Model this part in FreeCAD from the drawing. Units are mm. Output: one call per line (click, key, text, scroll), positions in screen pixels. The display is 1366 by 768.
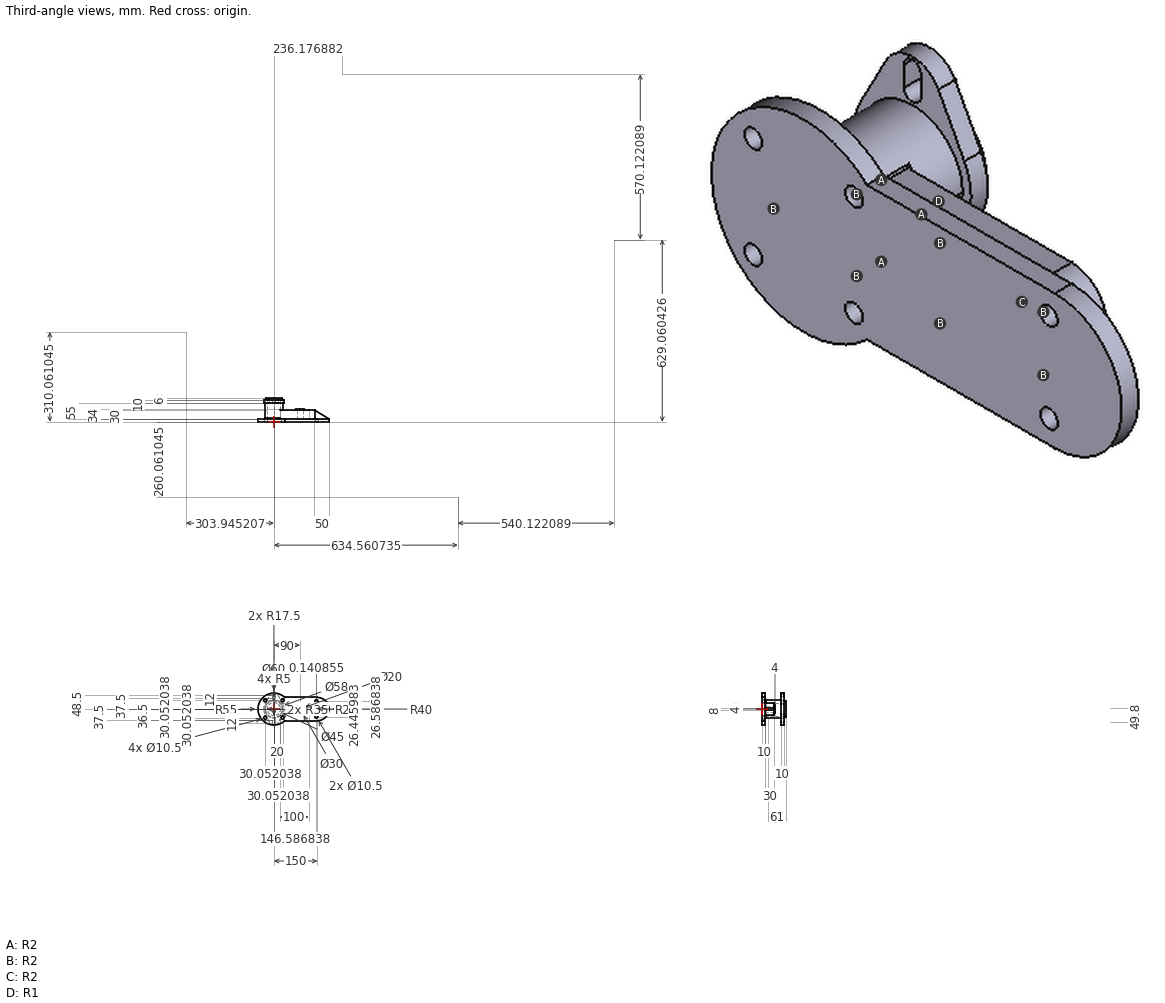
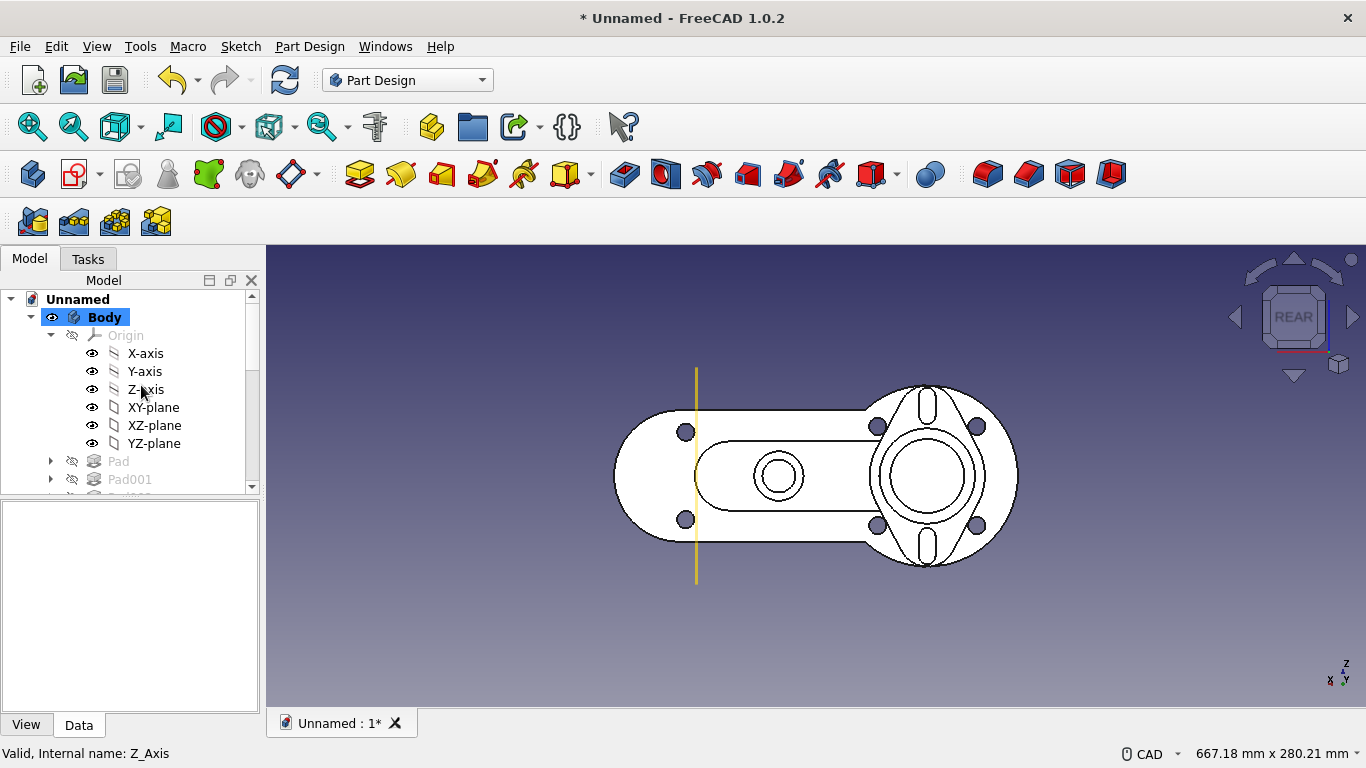
scroll(101, 385, down, 6)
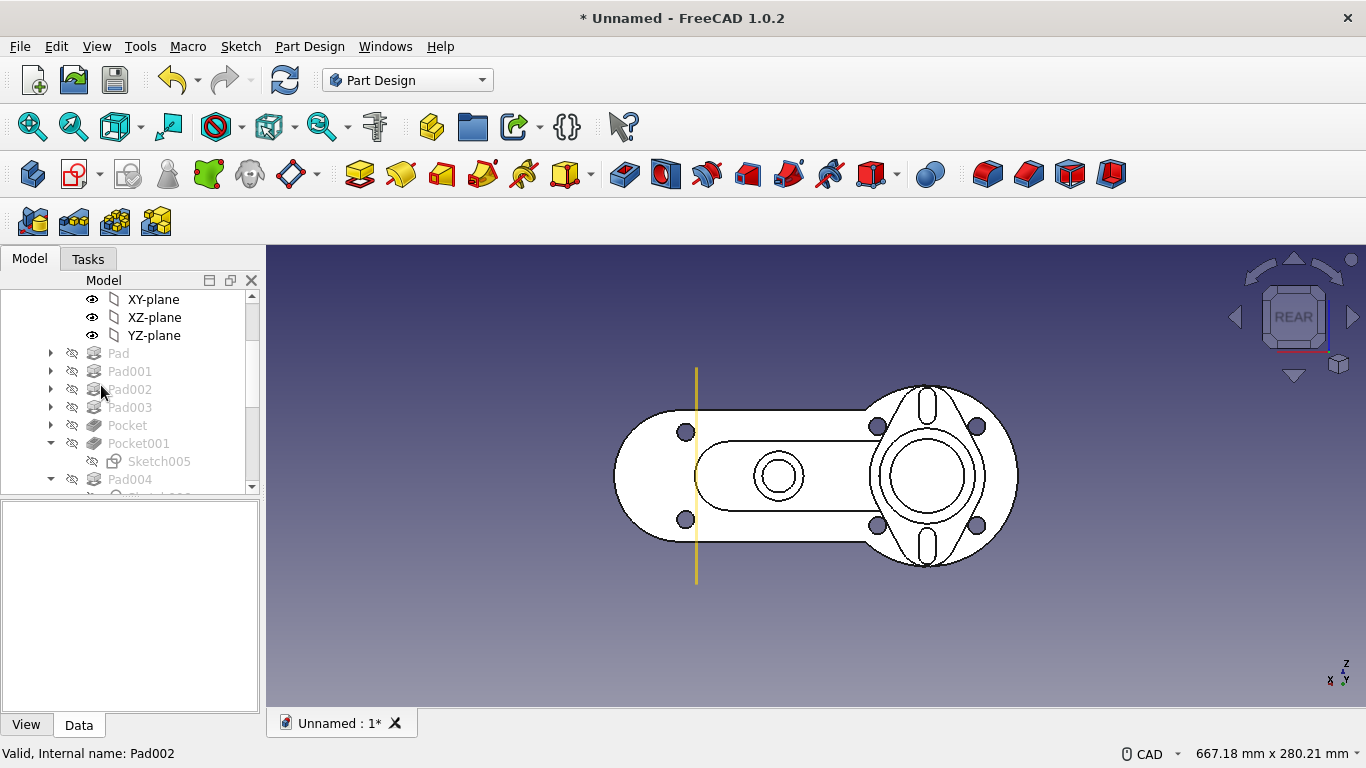
click(117, 479)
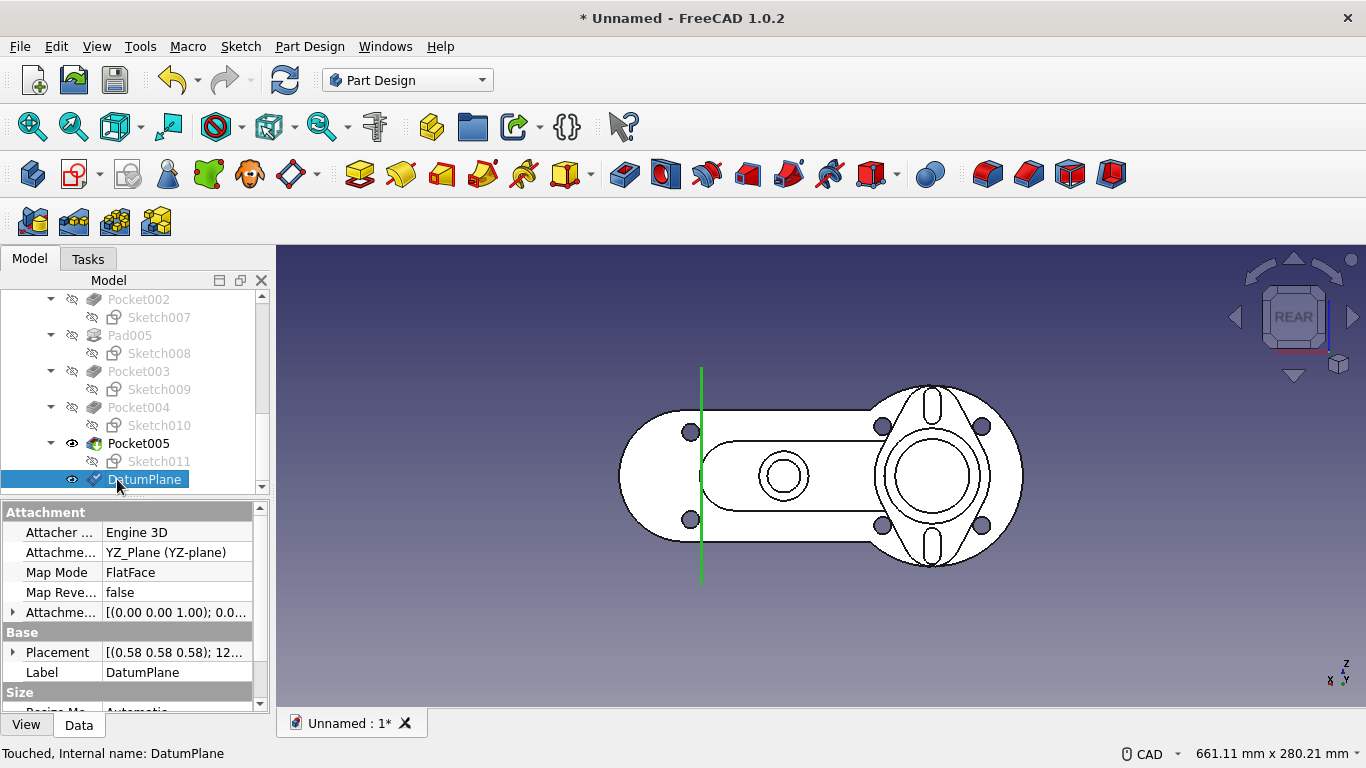
click(74, 174)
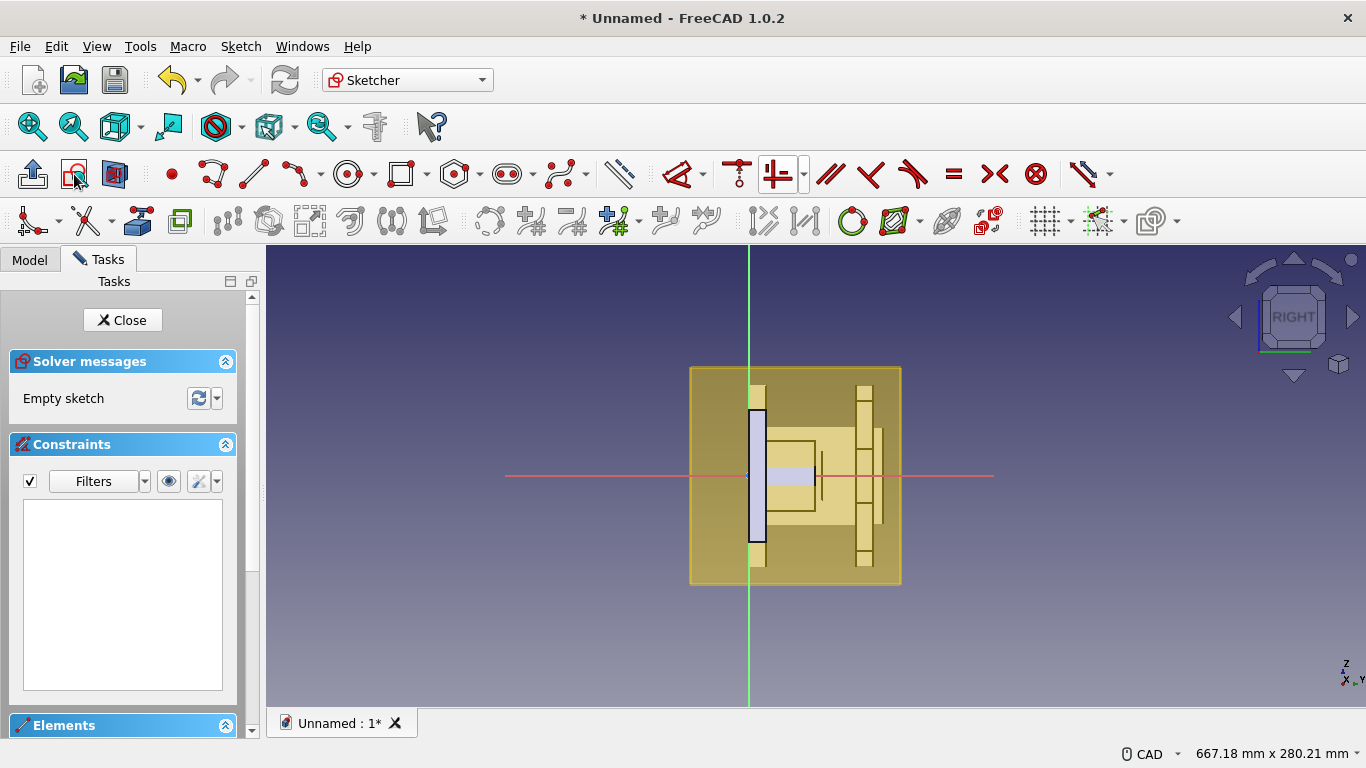
key(q)
key(s)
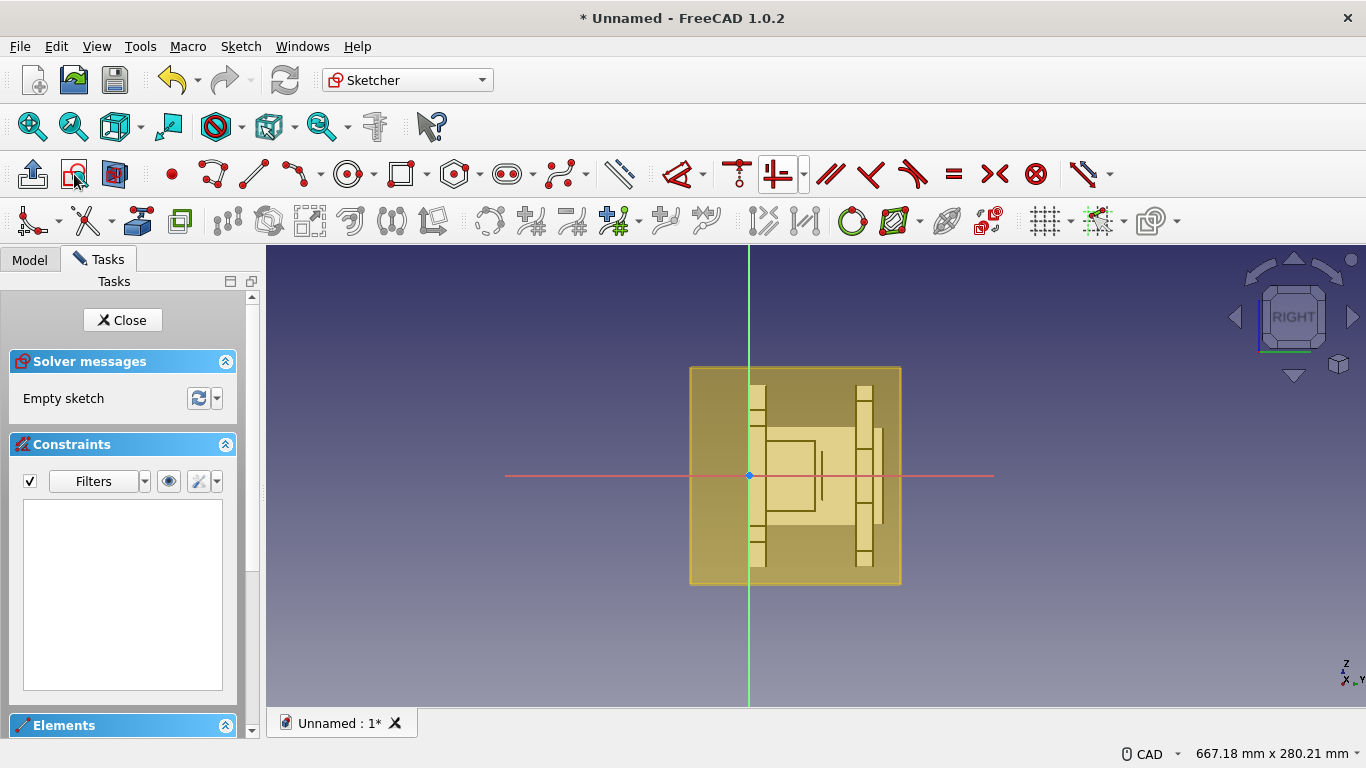
scroll(787, 476, up, 11)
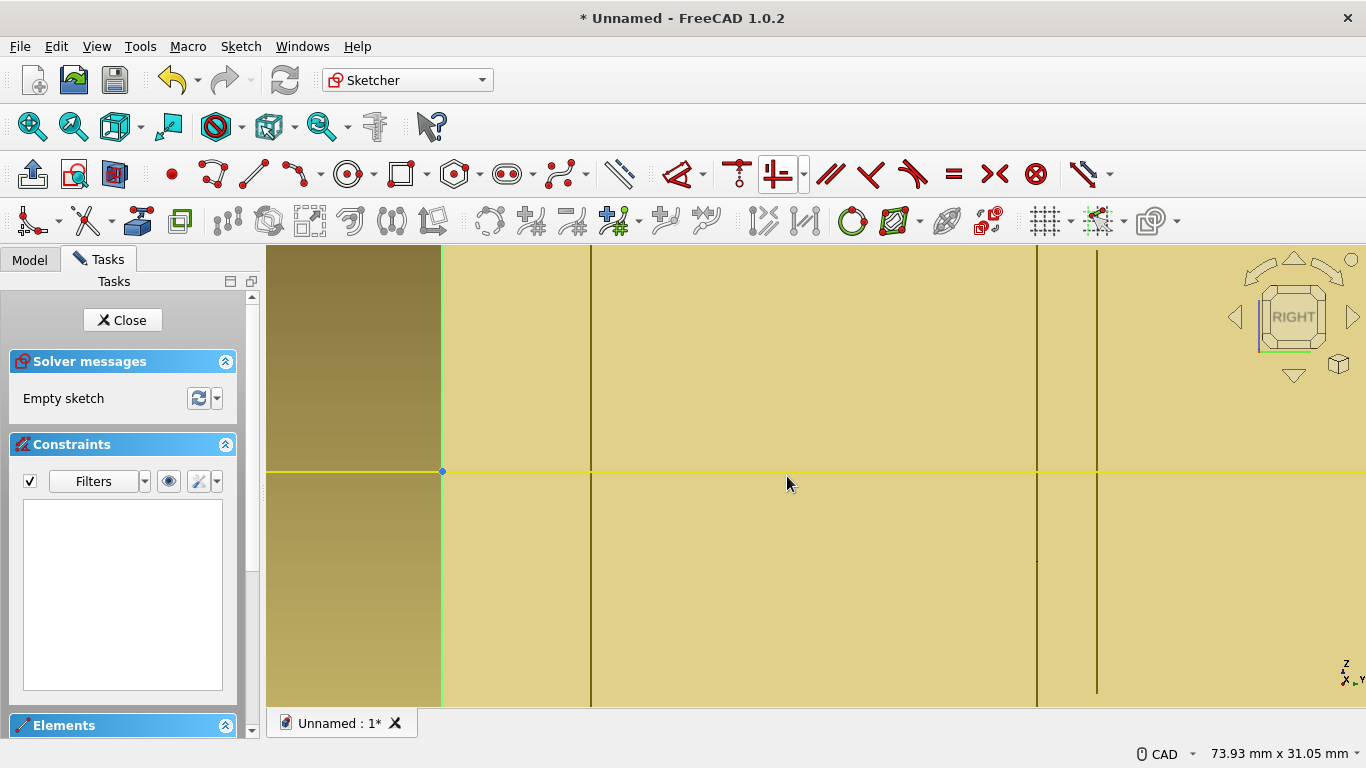
key(g)
key(r)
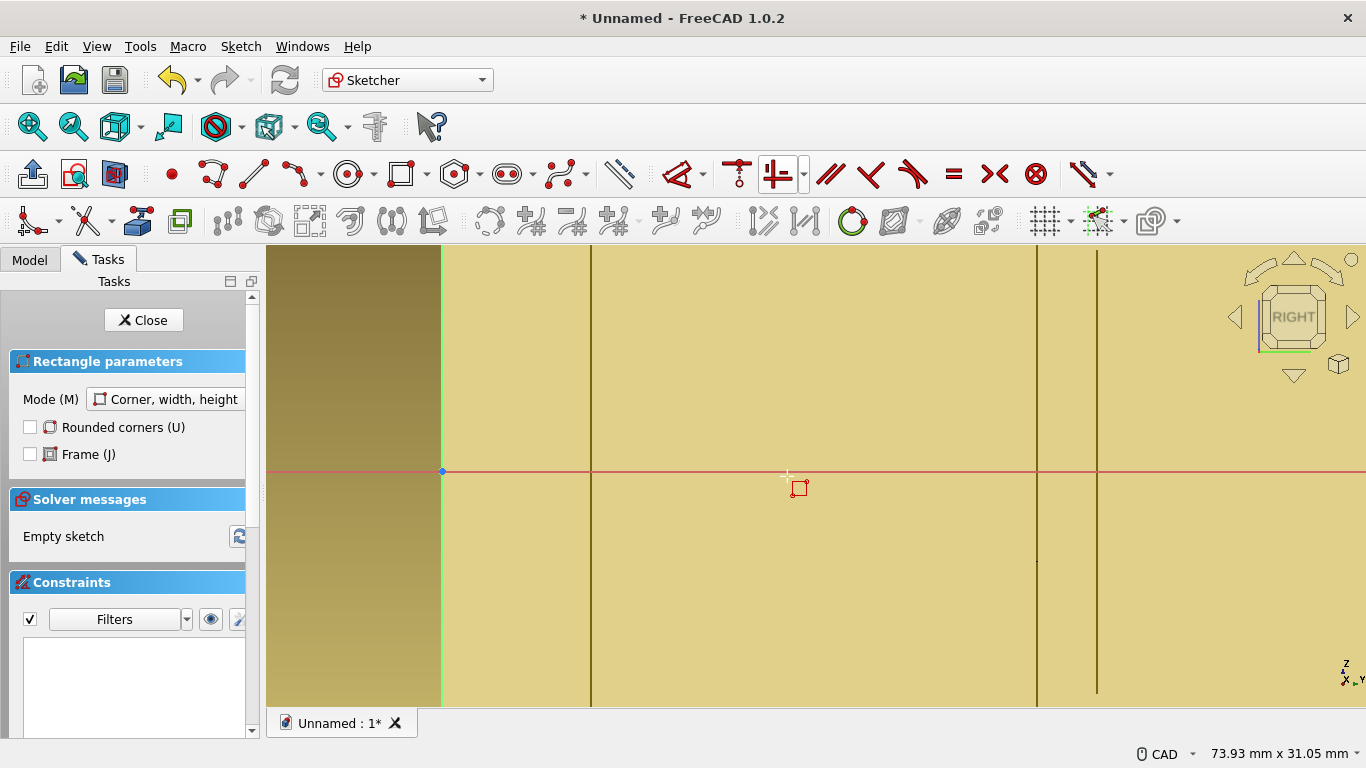
click(591, 412)
click(1037, 531)
key(Escape)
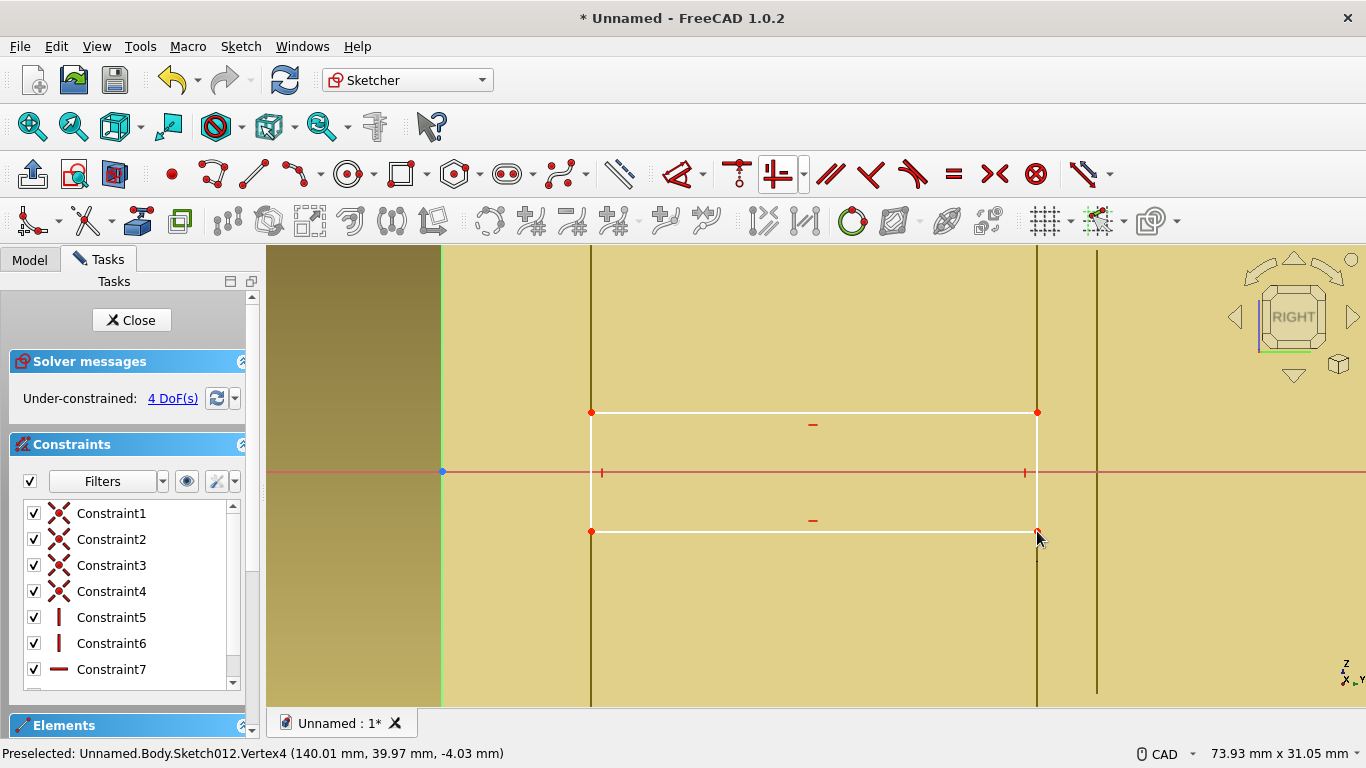
key(d)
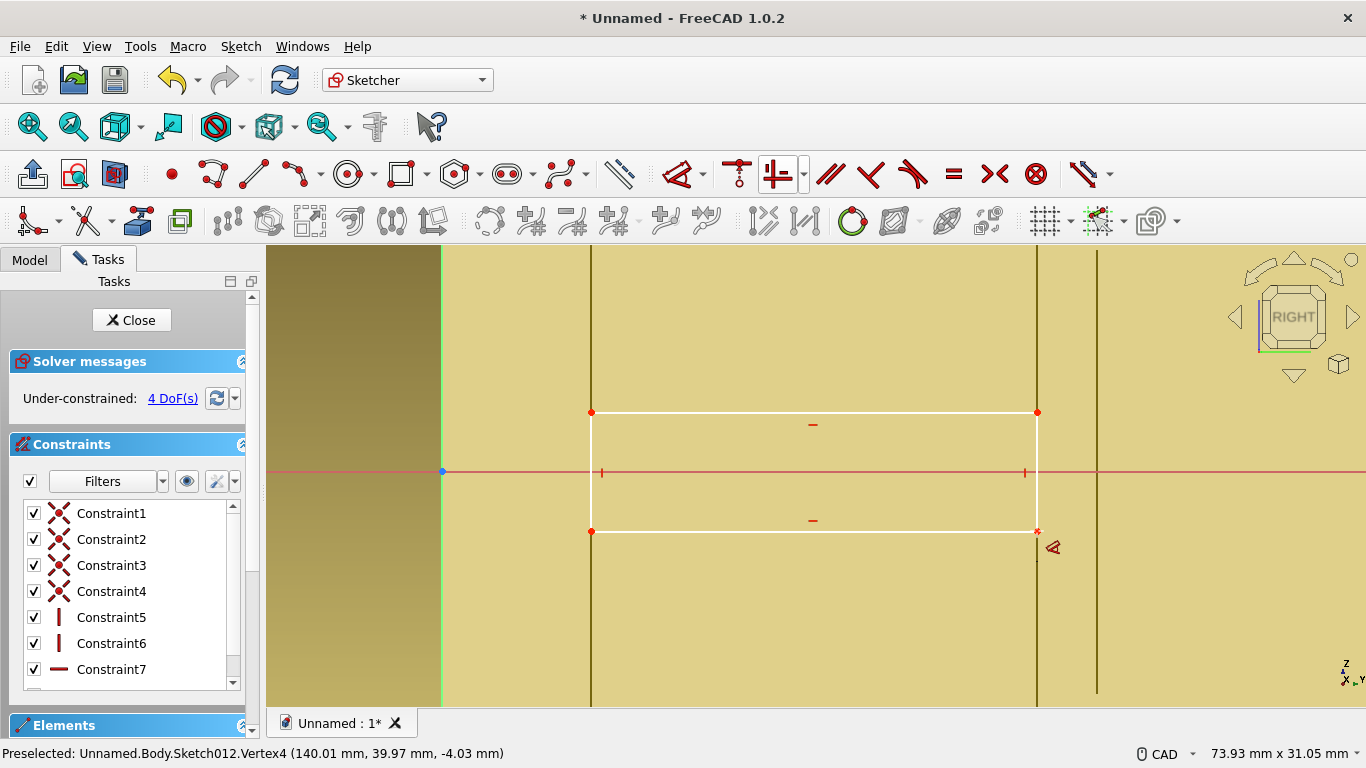
click(591, 449)
click(557, 445)